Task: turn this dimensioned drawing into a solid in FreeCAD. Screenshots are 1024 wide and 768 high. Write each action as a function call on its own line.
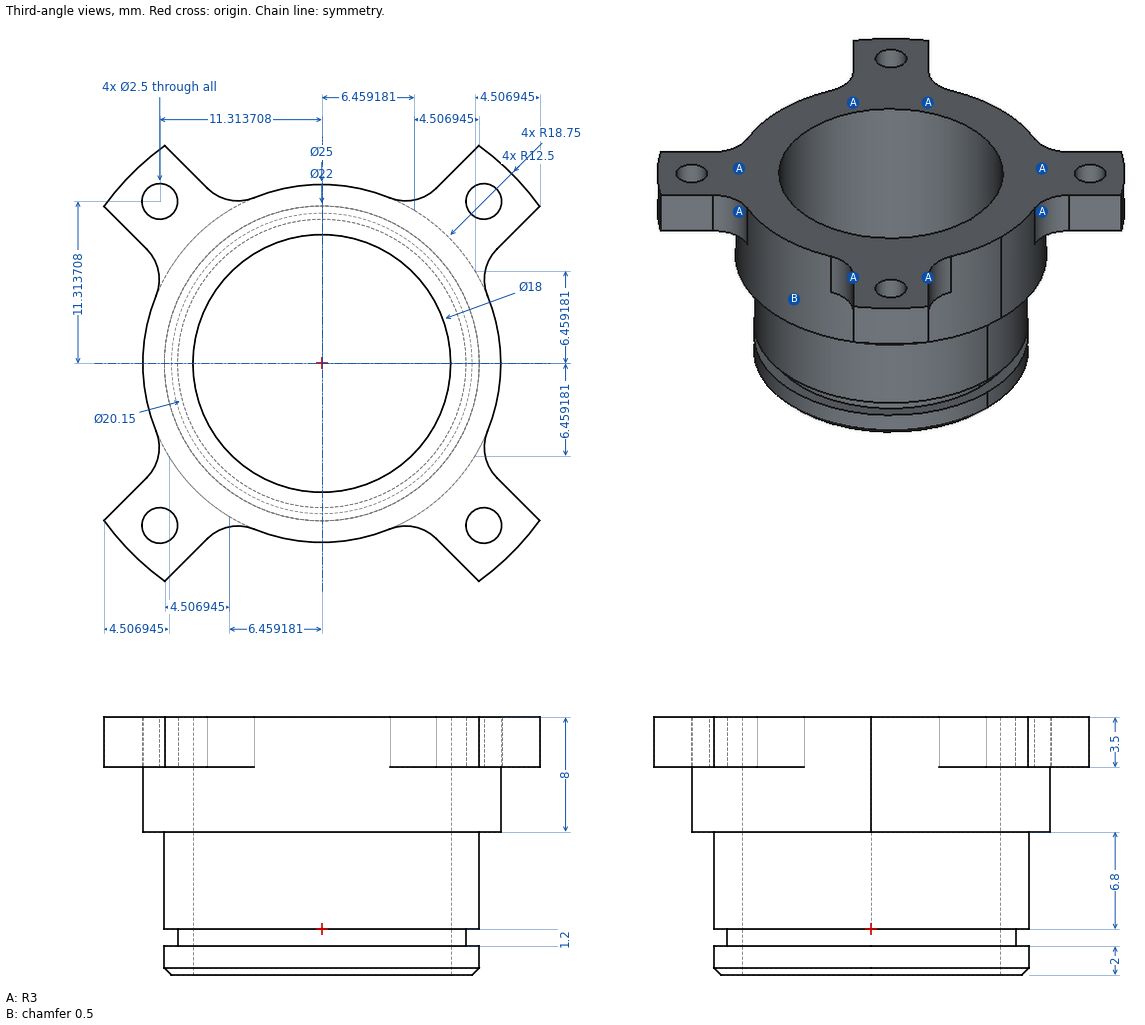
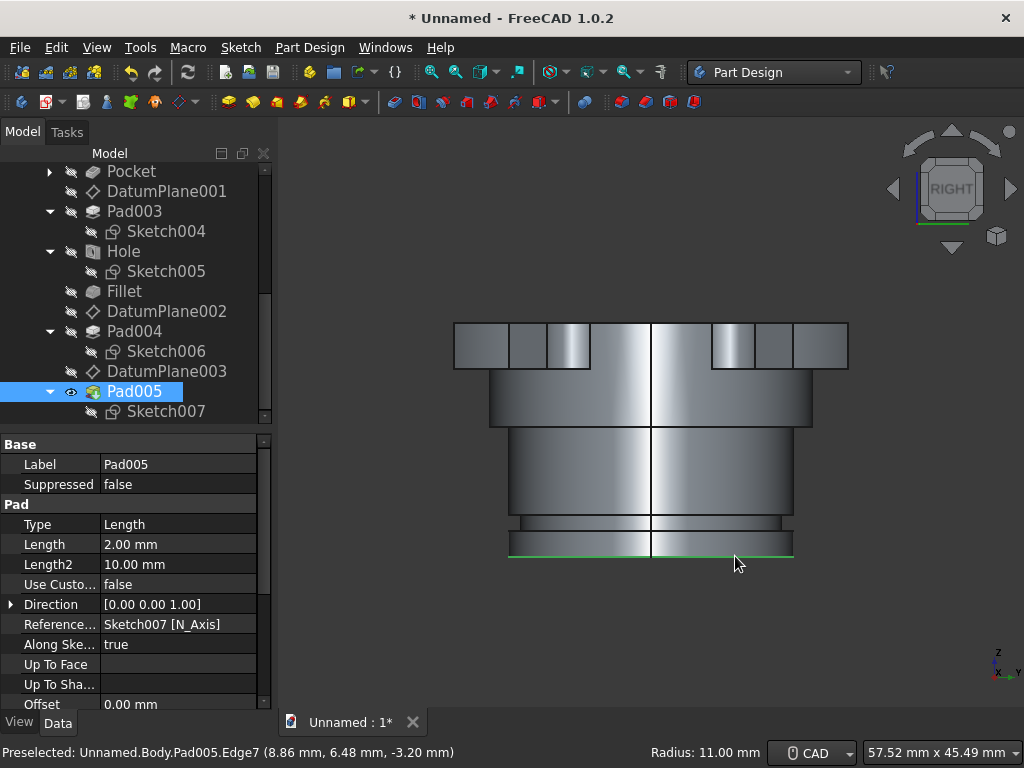
click(646, 102)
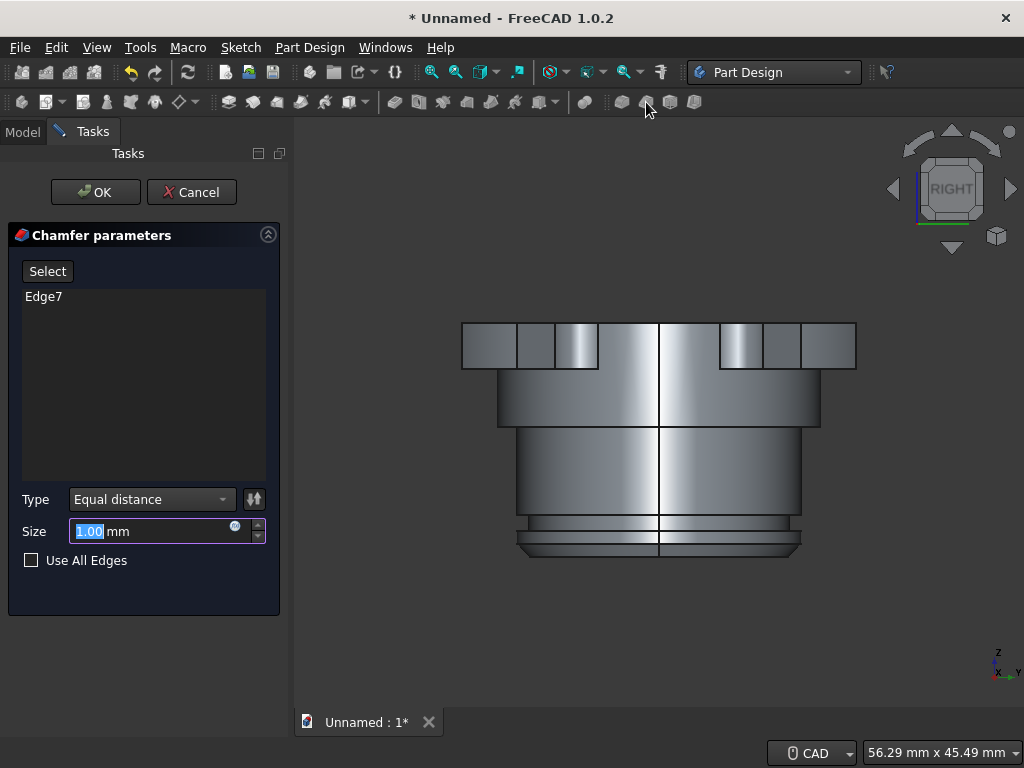
text(0.5)
key(Tab)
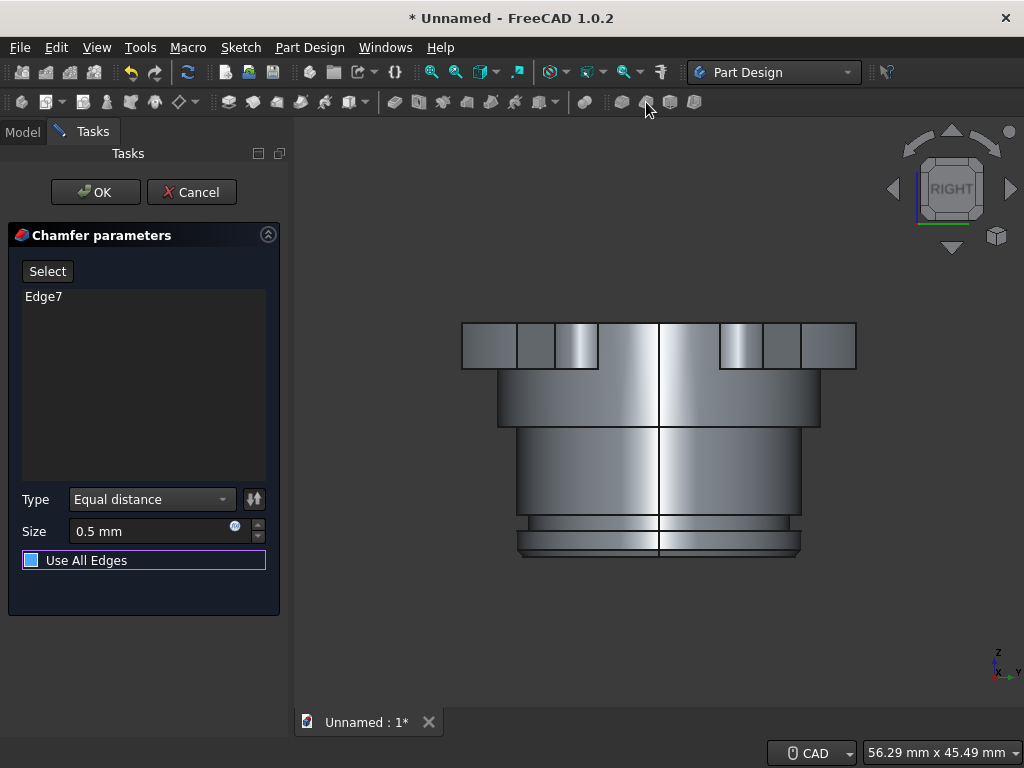
click(96, 192)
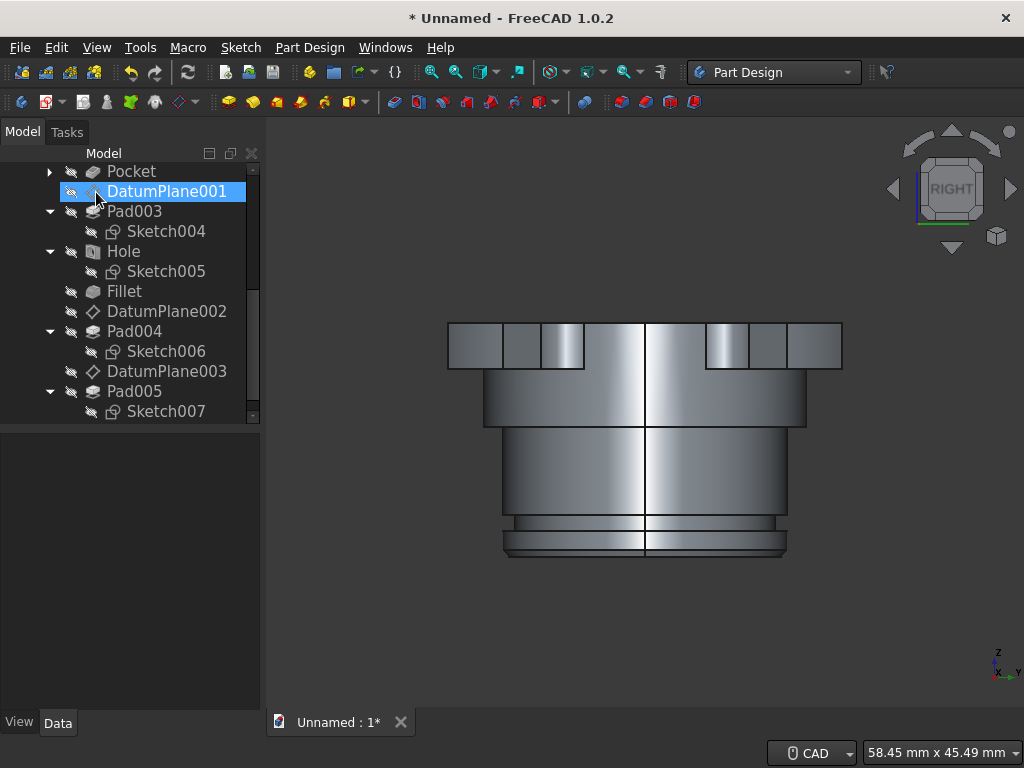
key(0)